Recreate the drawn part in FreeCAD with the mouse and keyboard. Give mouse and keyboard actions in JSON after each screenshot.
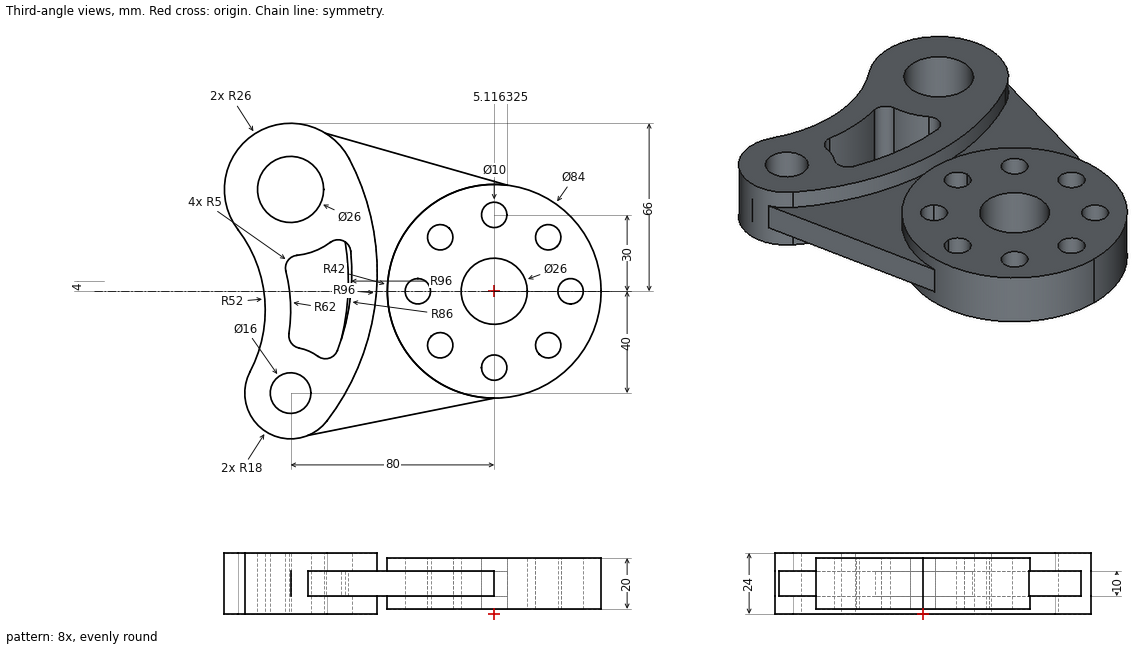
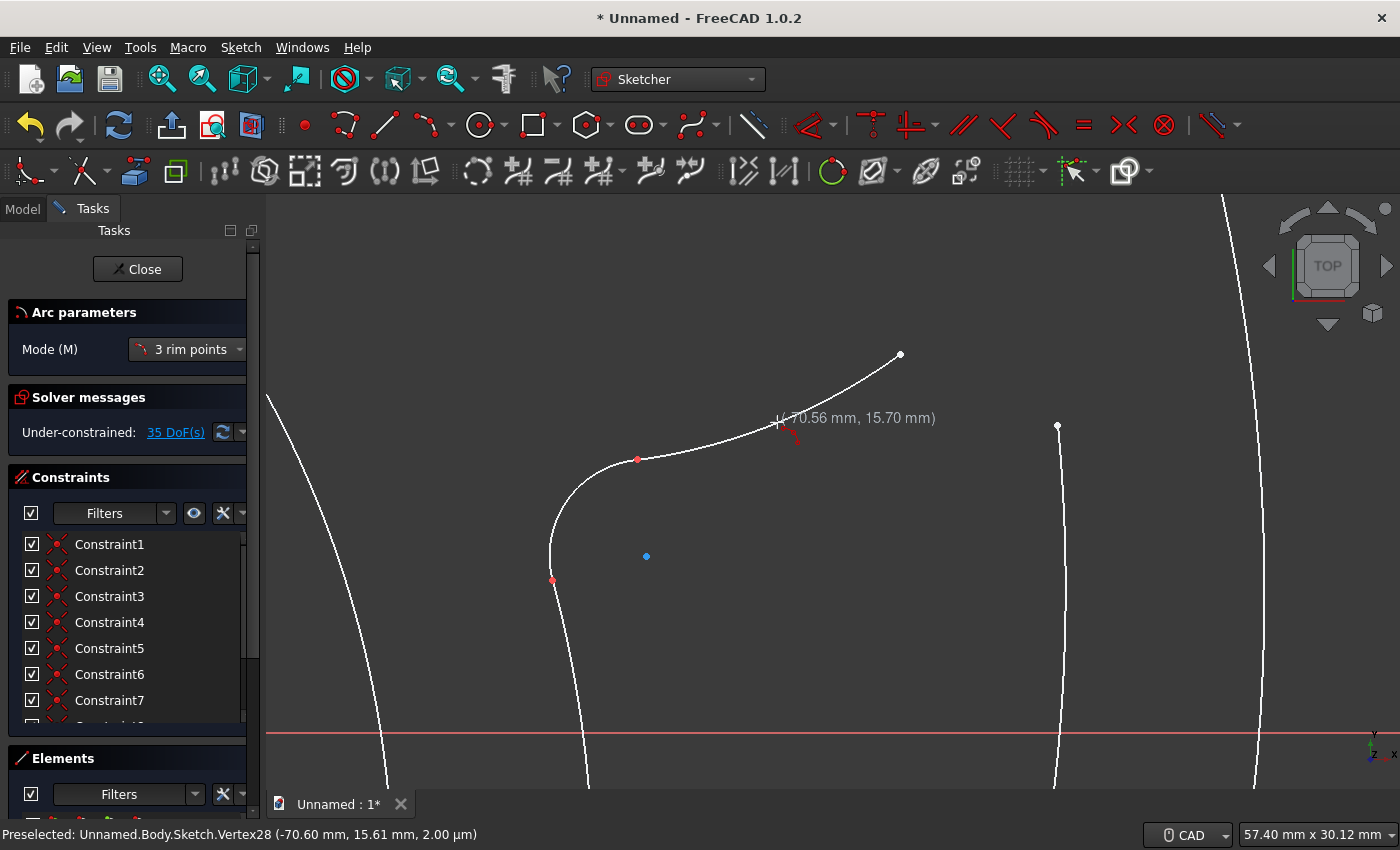
{"action": "scroll", "coordinate": [683, 457], "scroll_direction": "down", "scroll_amount": 9}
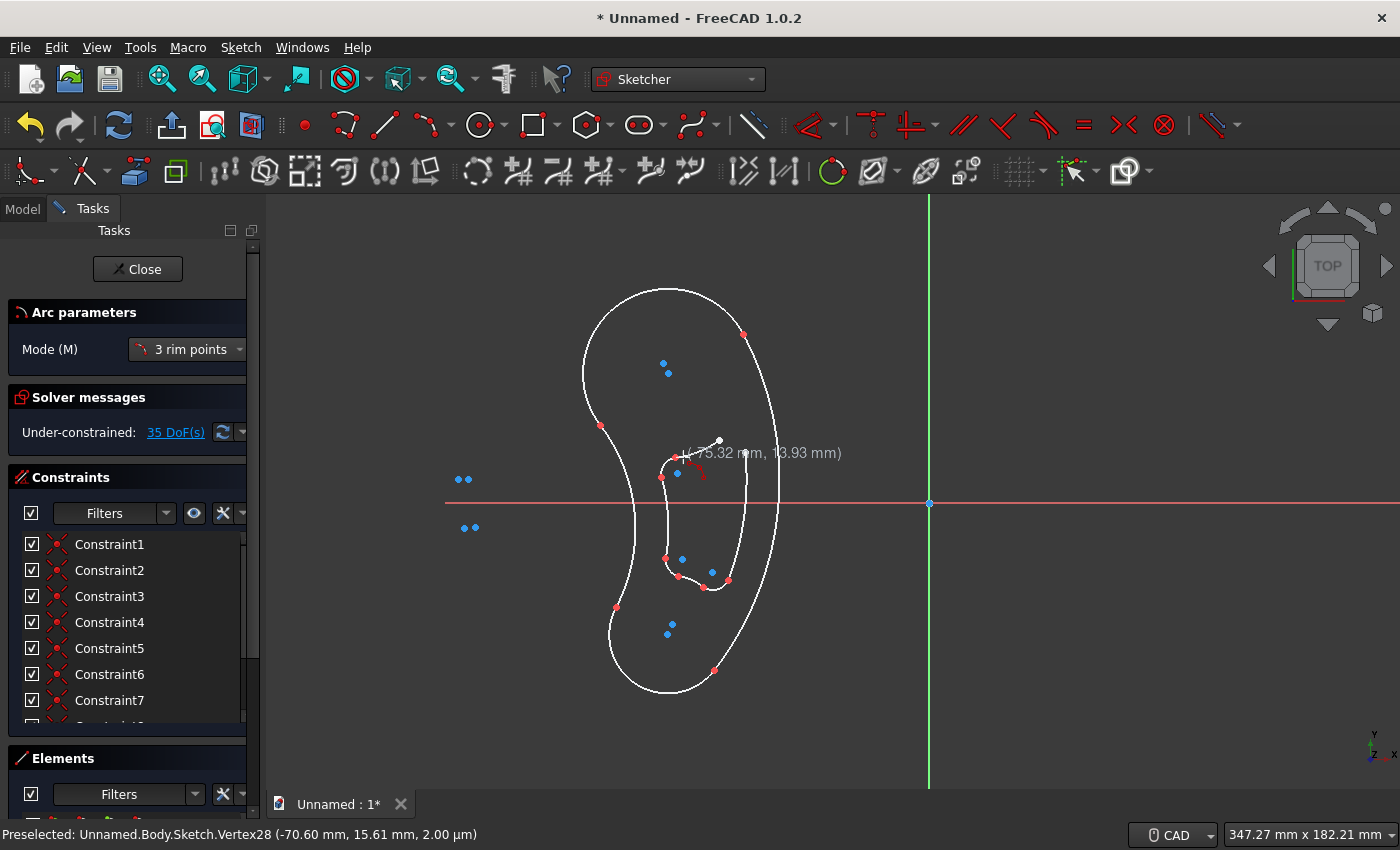
{"action": "left_click", "coordinate": [719, 440]}
{"action": "left_click", "coordinate": [745, 452]}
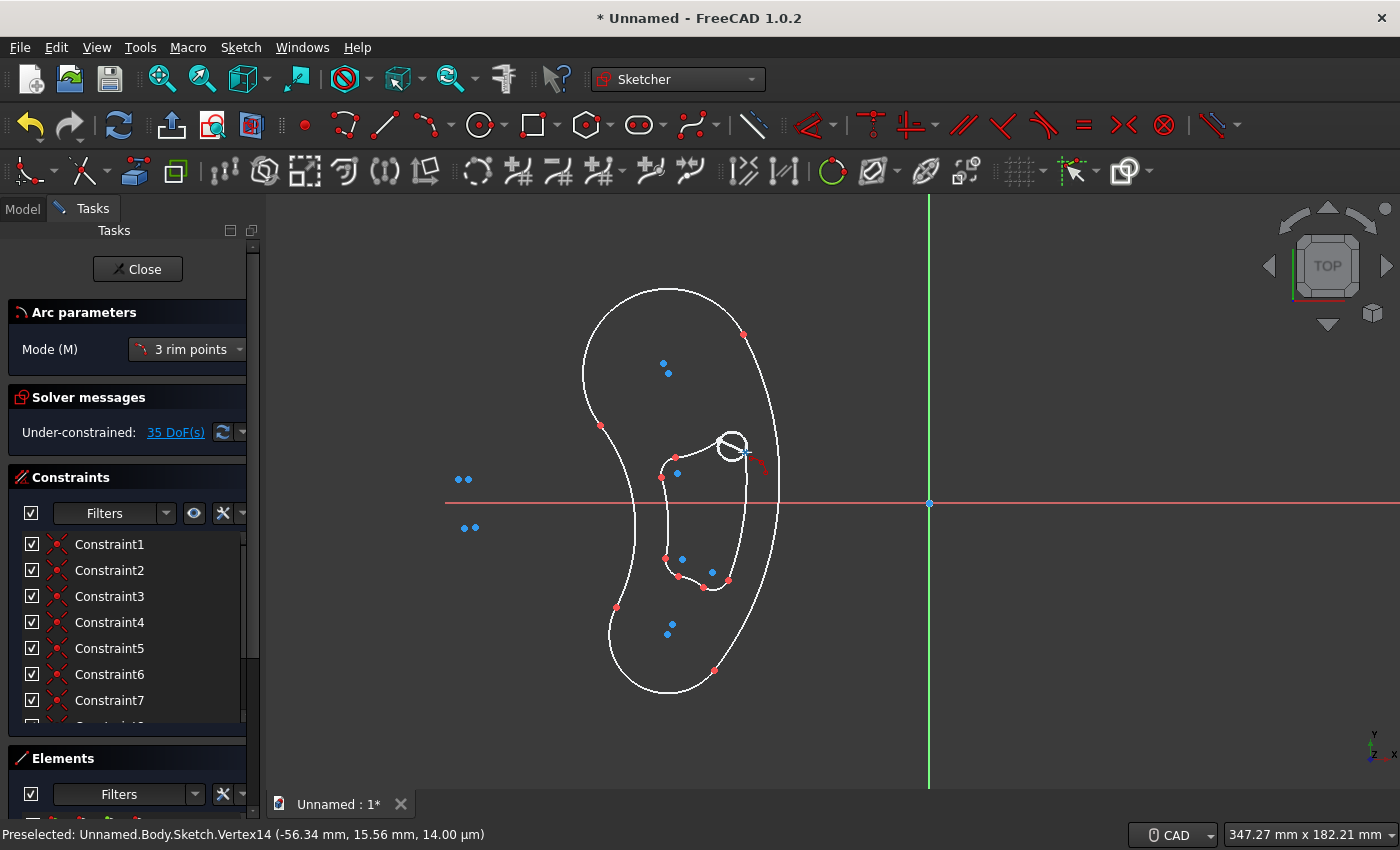
{"action": "scroll", "coordinate": [736, 438], "scroll_direction": "up", "scroll_amount": 4}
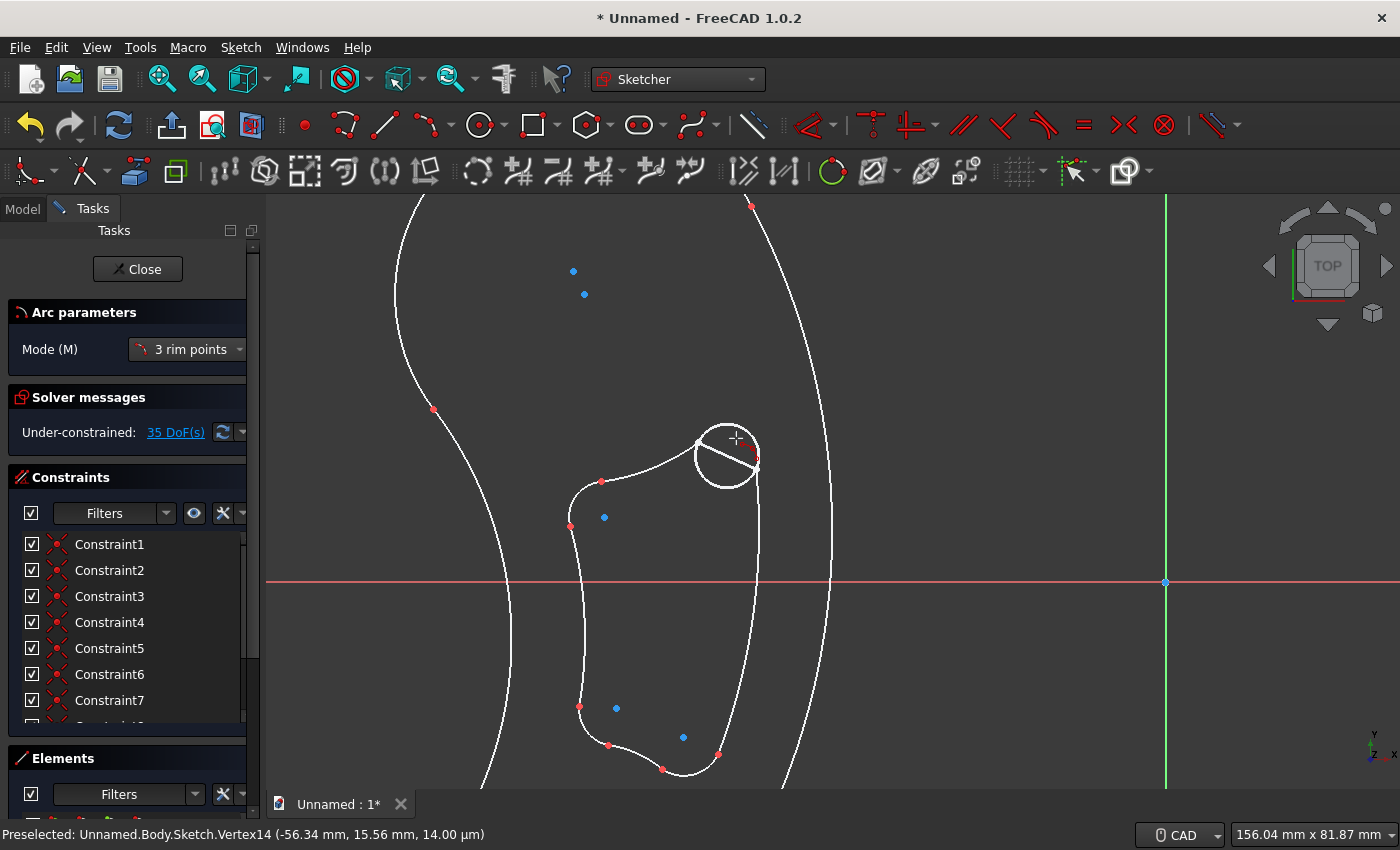
{"action": "left_click", "coordinate": [735, 438]}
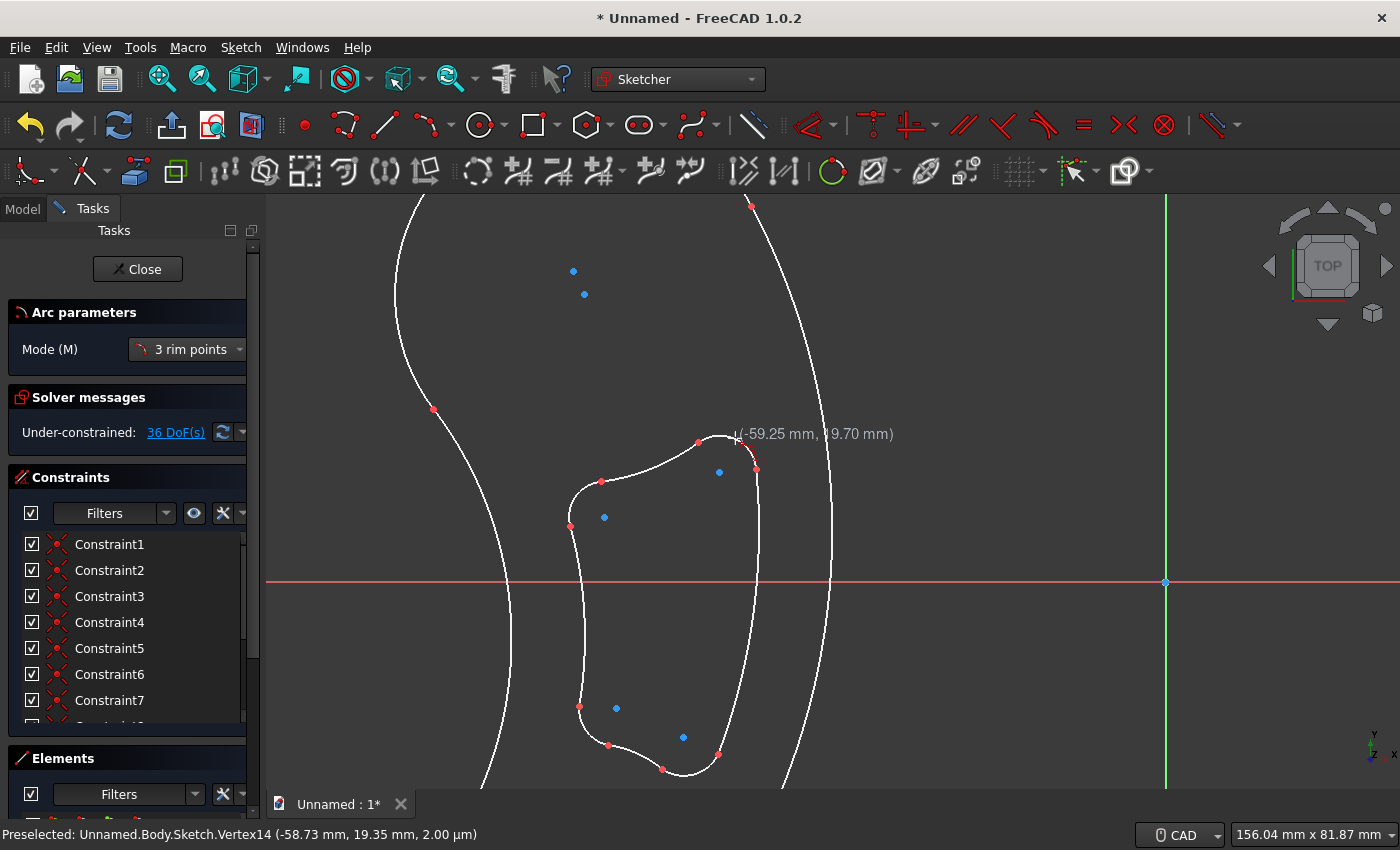
{"action": "left_click", "coordinate": [480, 126]}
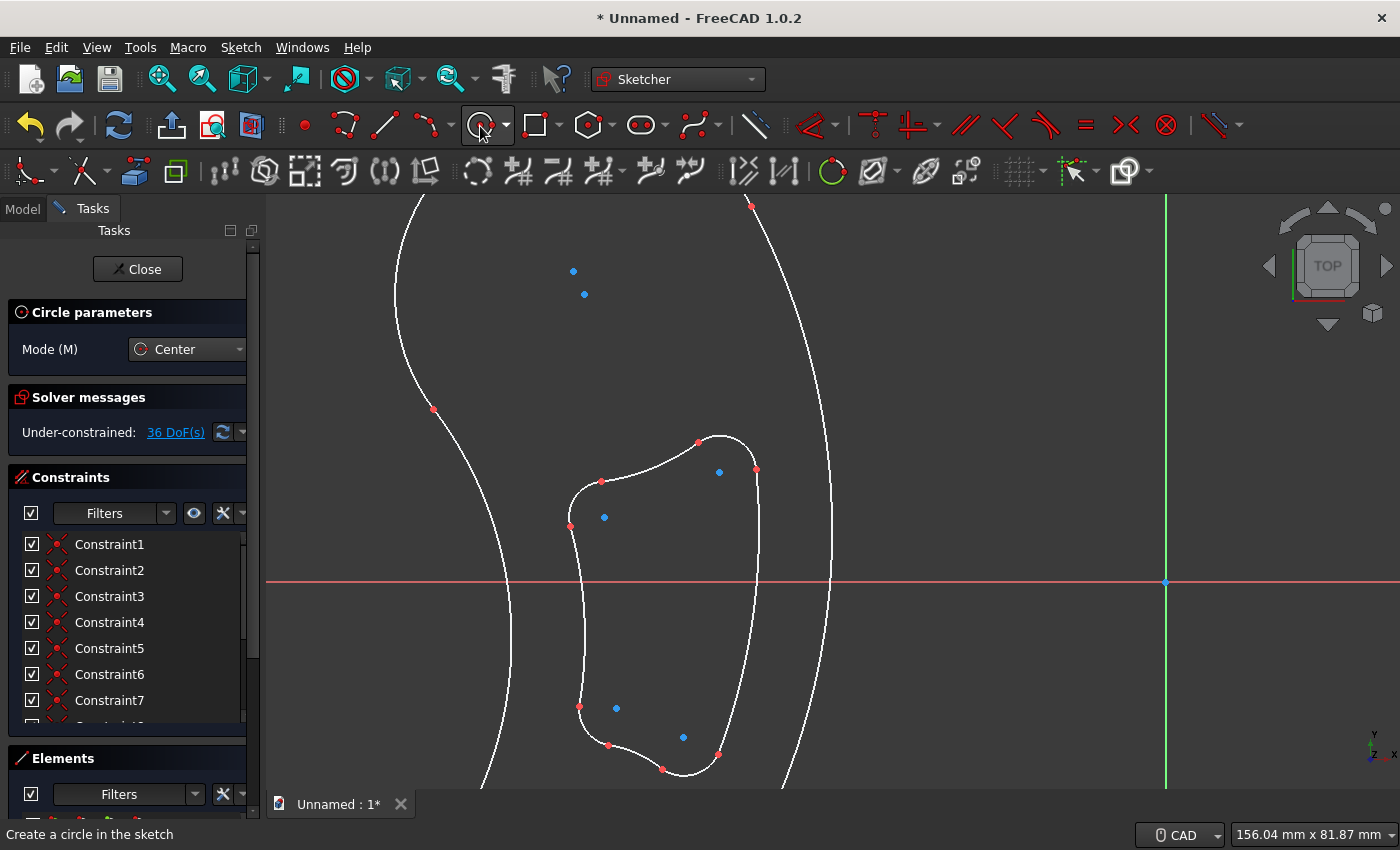
{"action": "scroll", "coordinate": [736, 437], "scroll_direction": "down", "scroll_amount": 4}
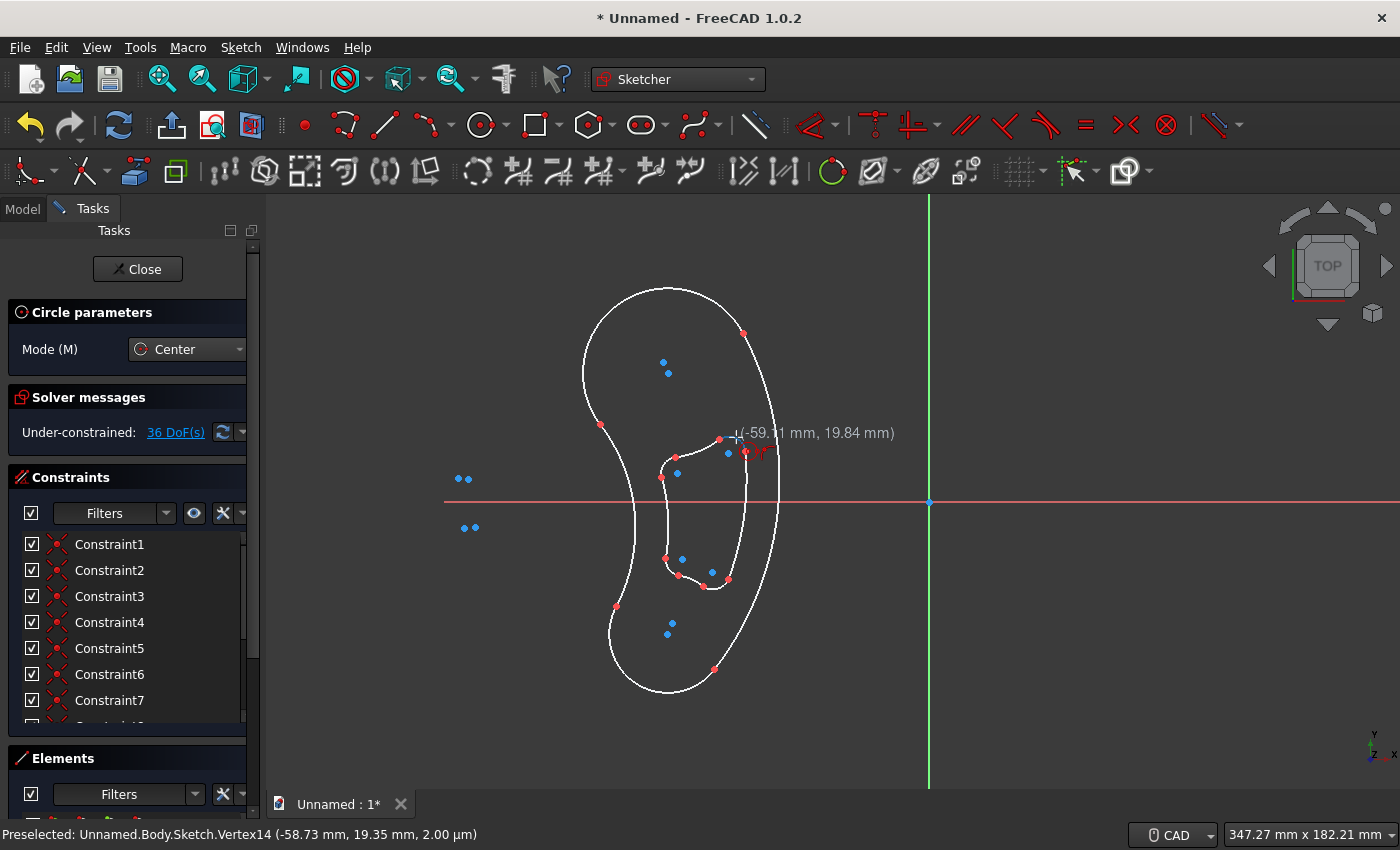
{"action": "left_click", "coordinate": [668, 633]}
{"action": "left_click", "coordinate": [686, 615]}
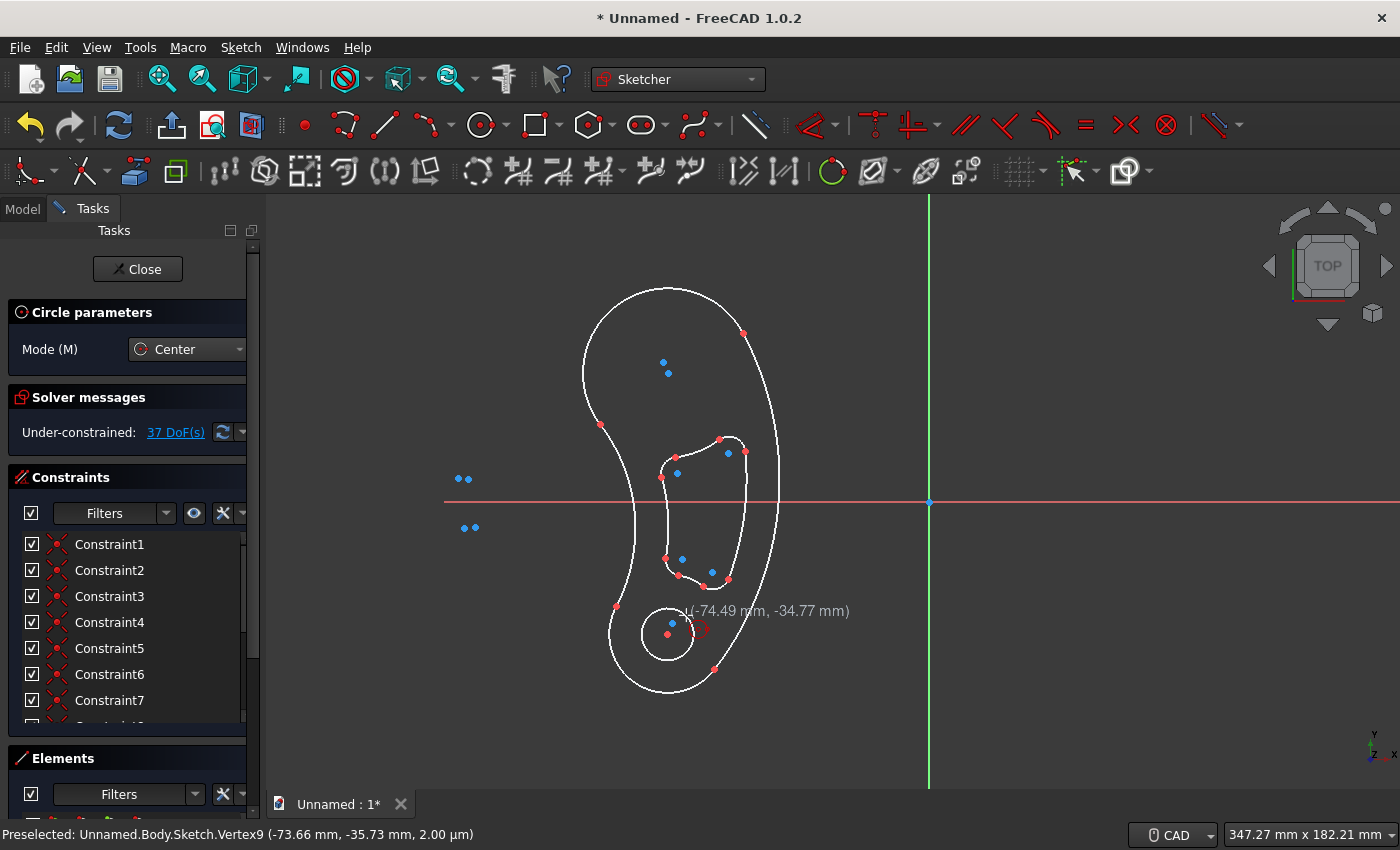
{"action": "left_click", "coordinate": [668, 372]}
{"action": "left_click", "coordinate": [698, 342]}
{"action": "key", "text": "Escape"}